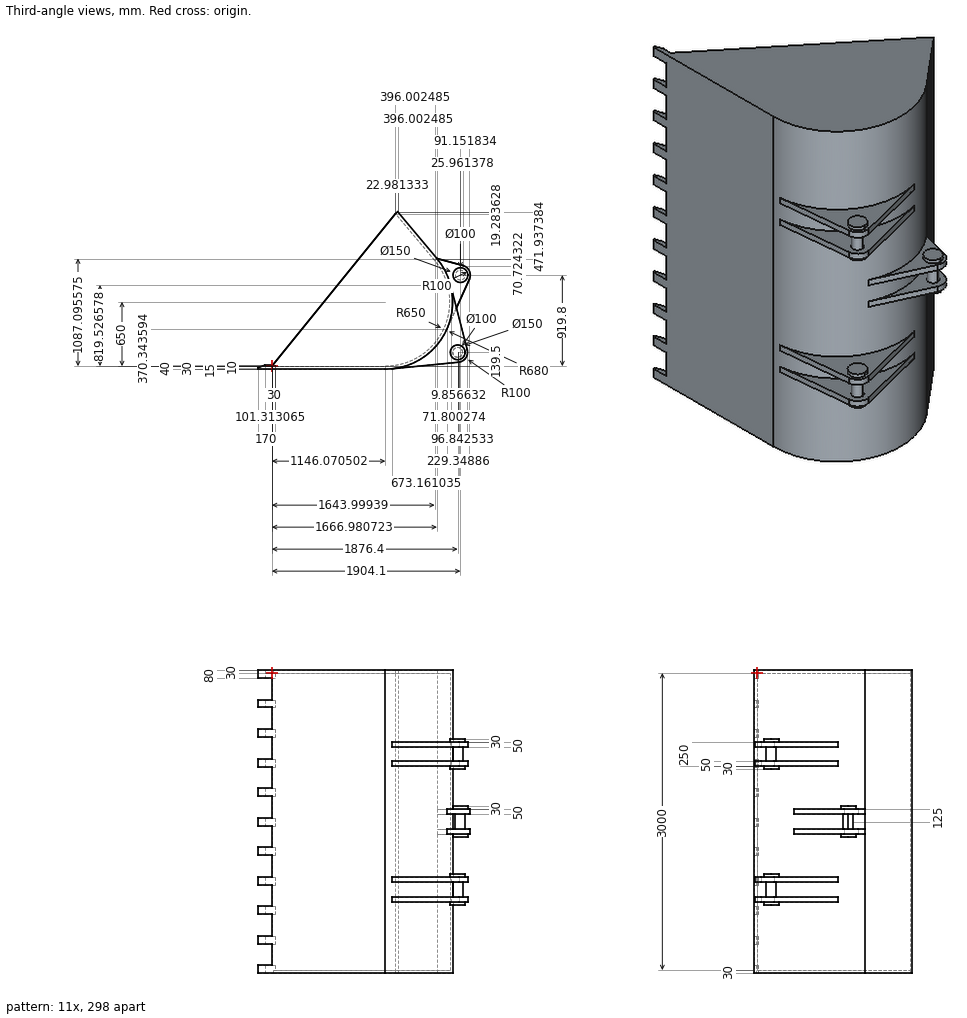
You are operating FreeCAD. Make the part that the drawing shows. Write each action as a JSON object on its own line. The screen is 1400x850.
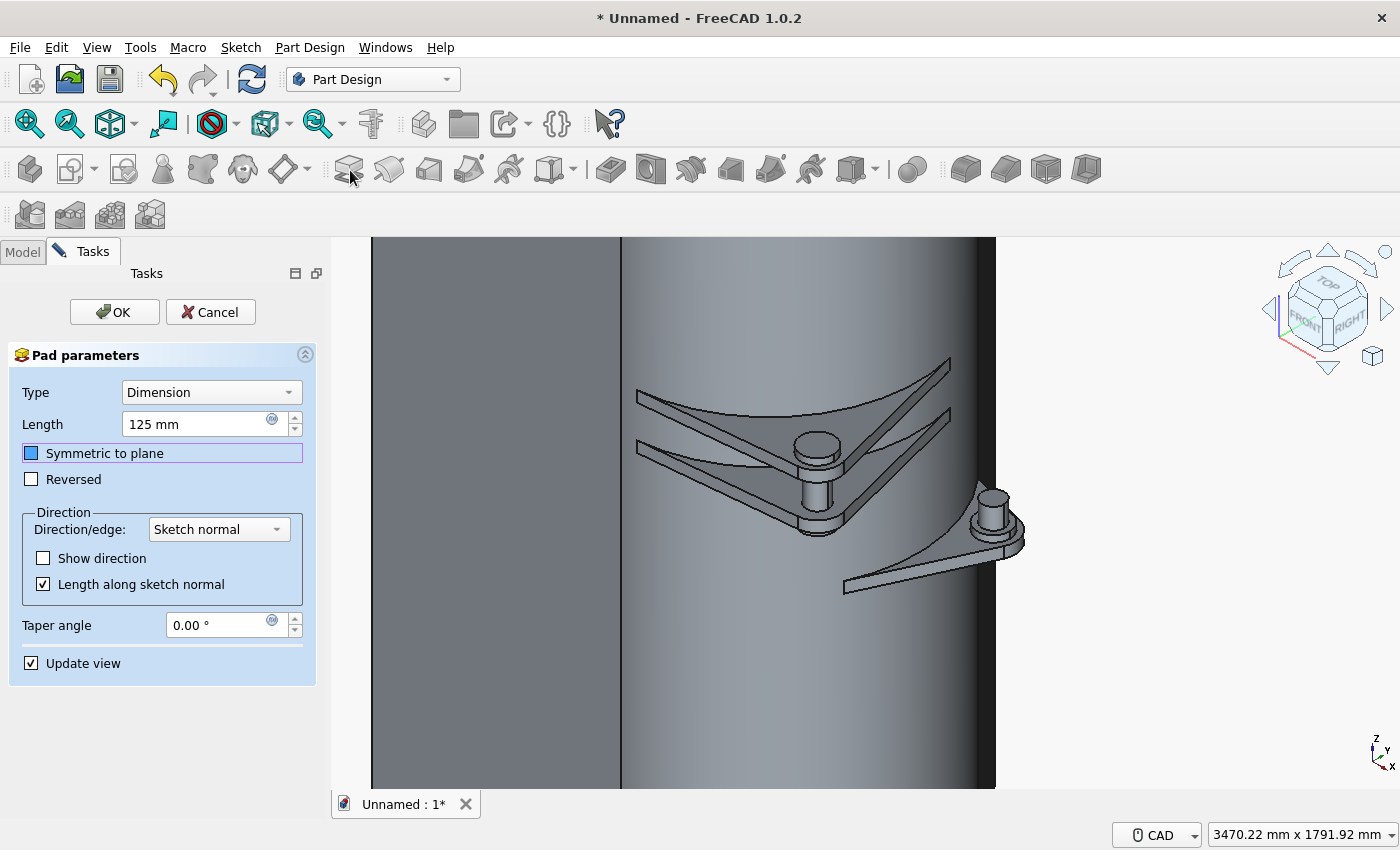
{"action": "left_click", "coordinate": [30, 479]}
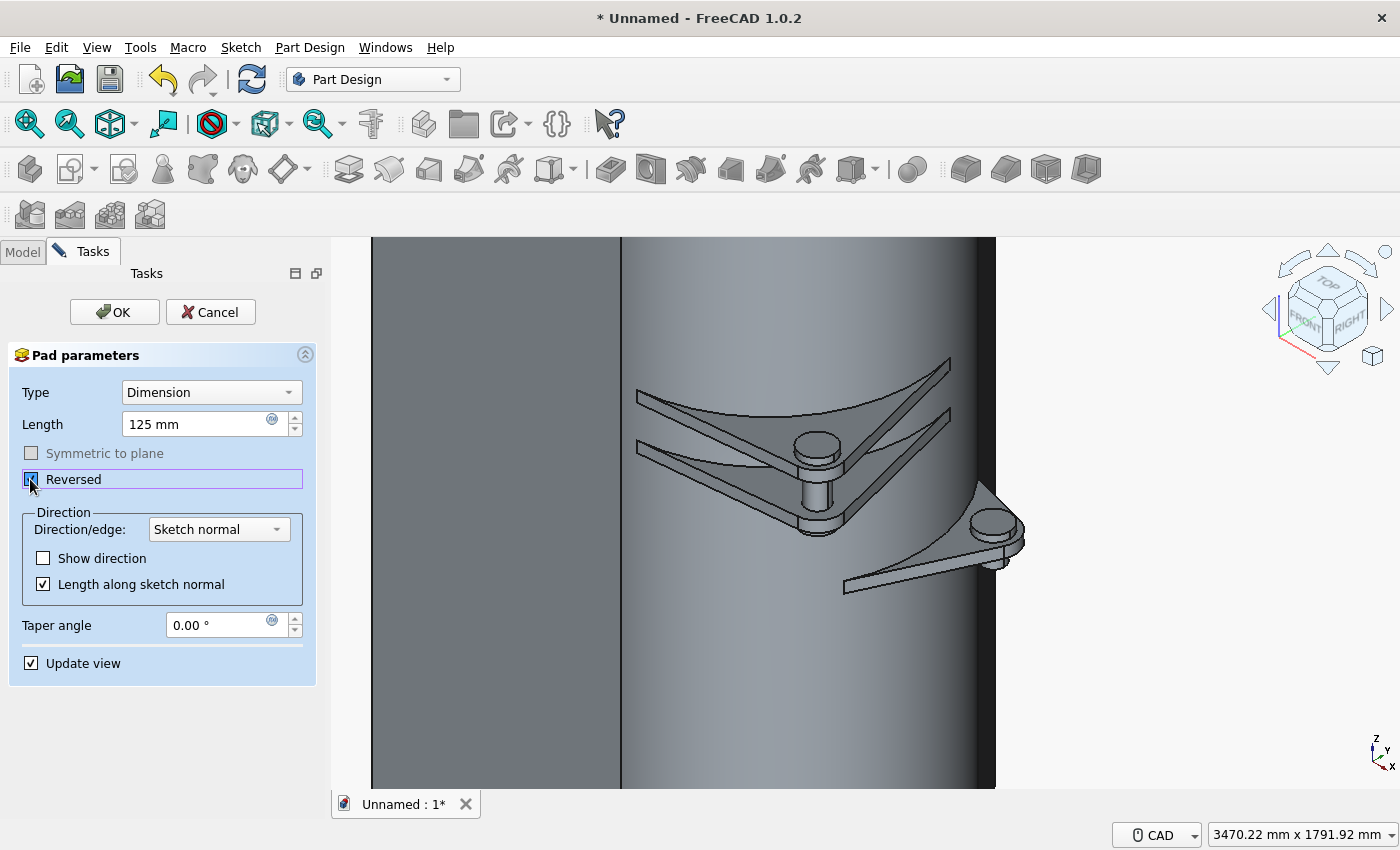
{"action": "left_click", "coordinate": [115, 312]}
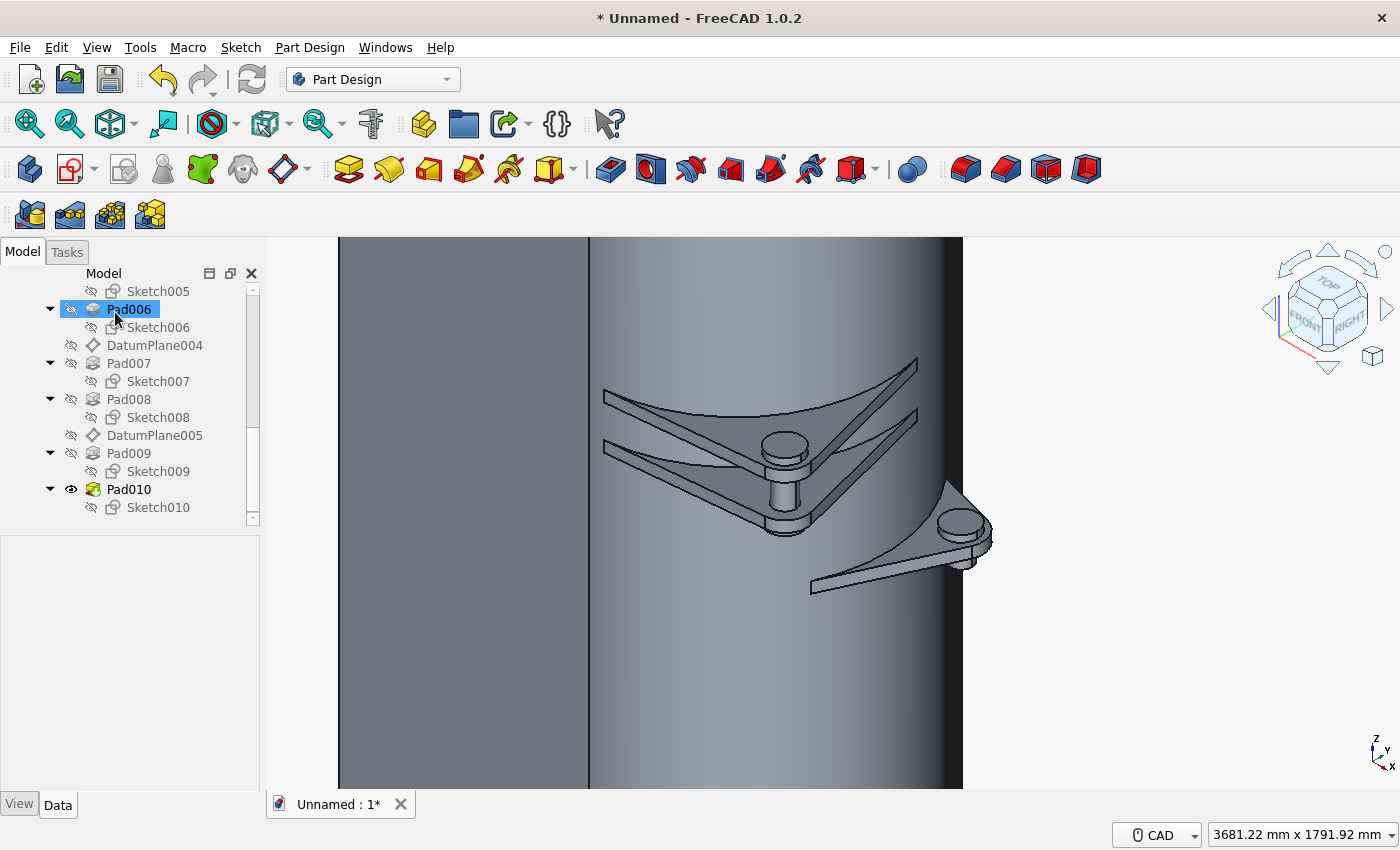
{"action": "key", "text": "v f"}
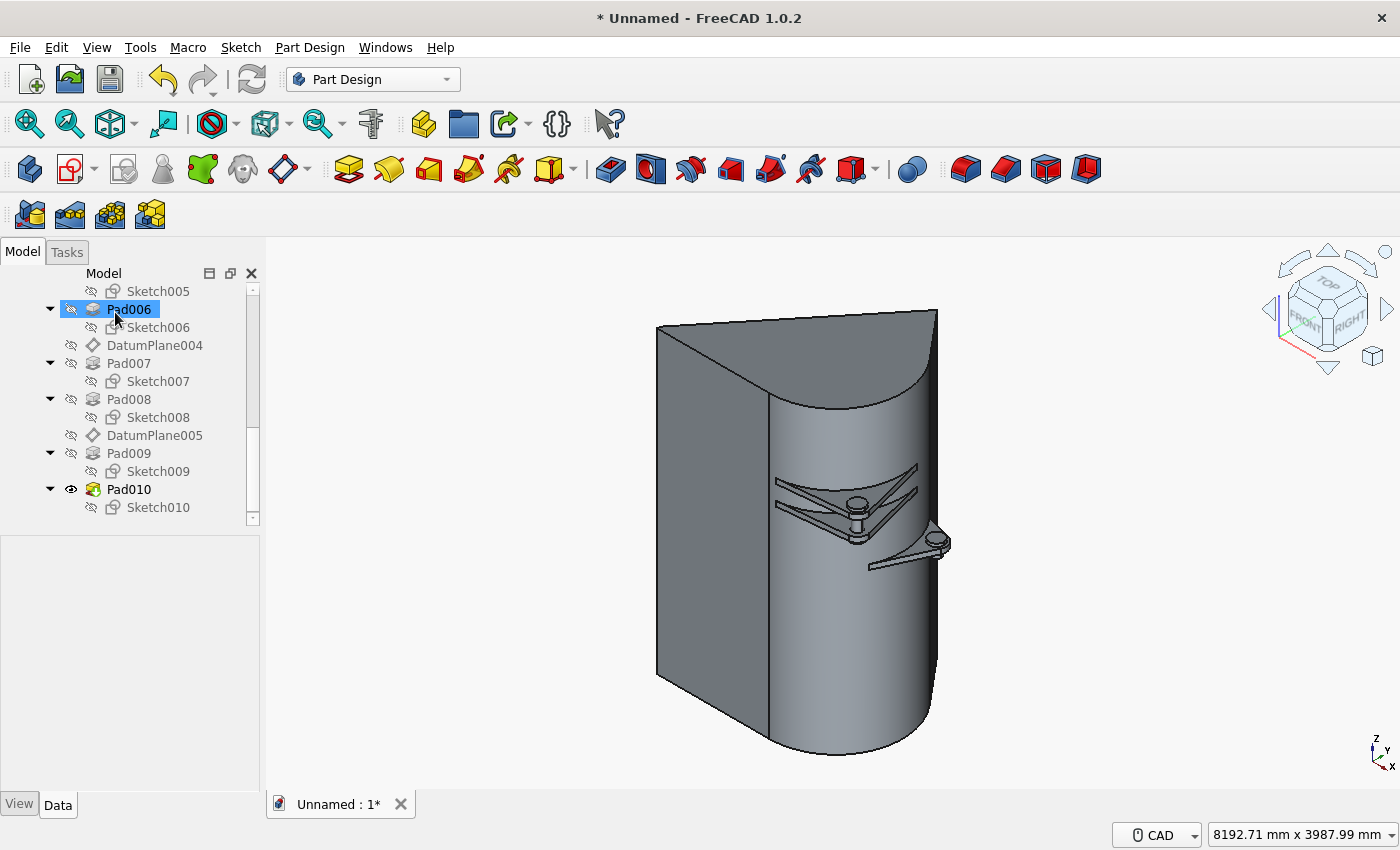
{"action": "scroll", "coordinate": [160, 395], "scroll_direction": "down", "scroll_amount": 3}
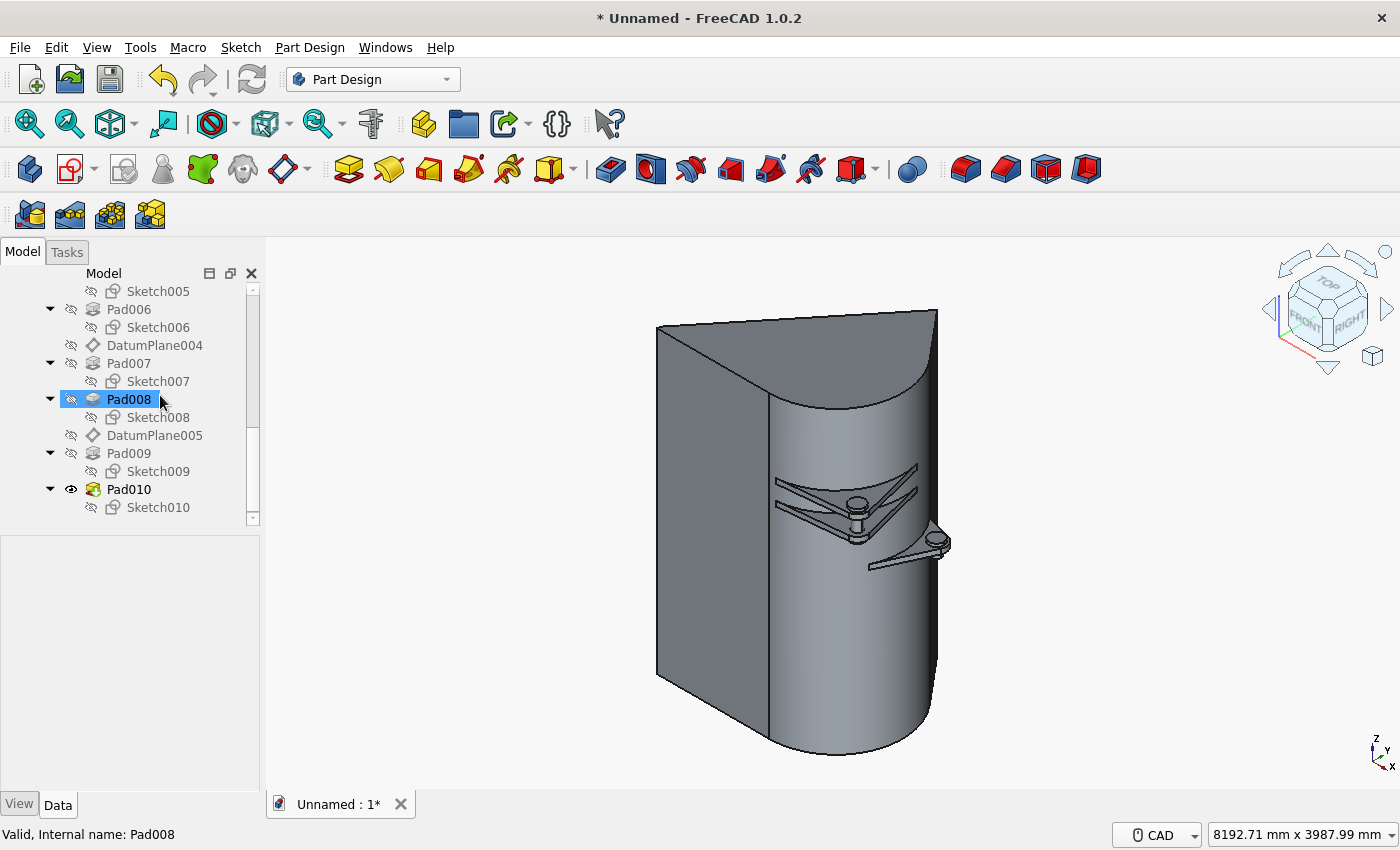
{"action": "scroll", "coordinate": [160, 395], "scroll_direction": "up", "scroll_amount": 15}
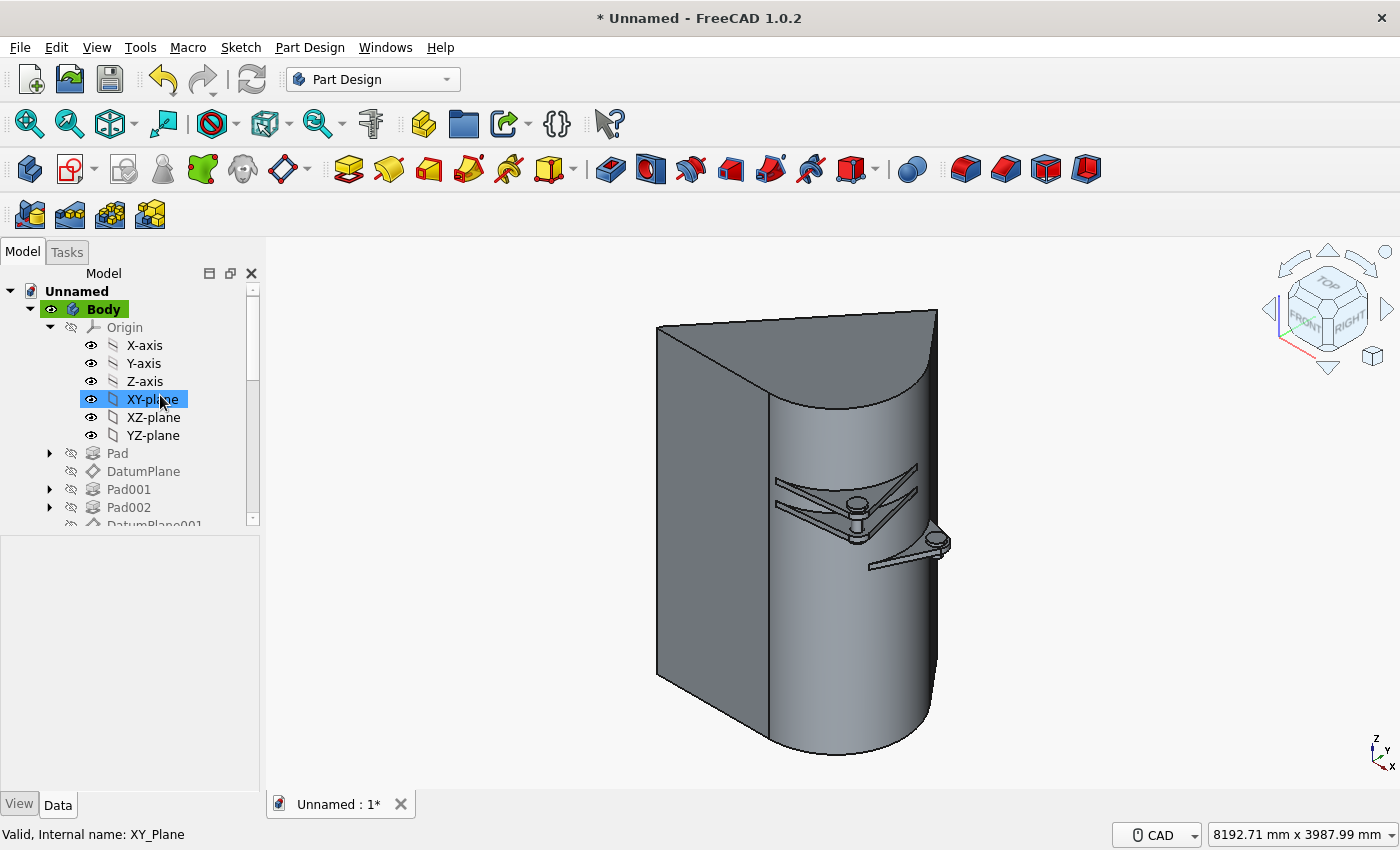
{"action": "left_click", "coordinate": [136, 399]}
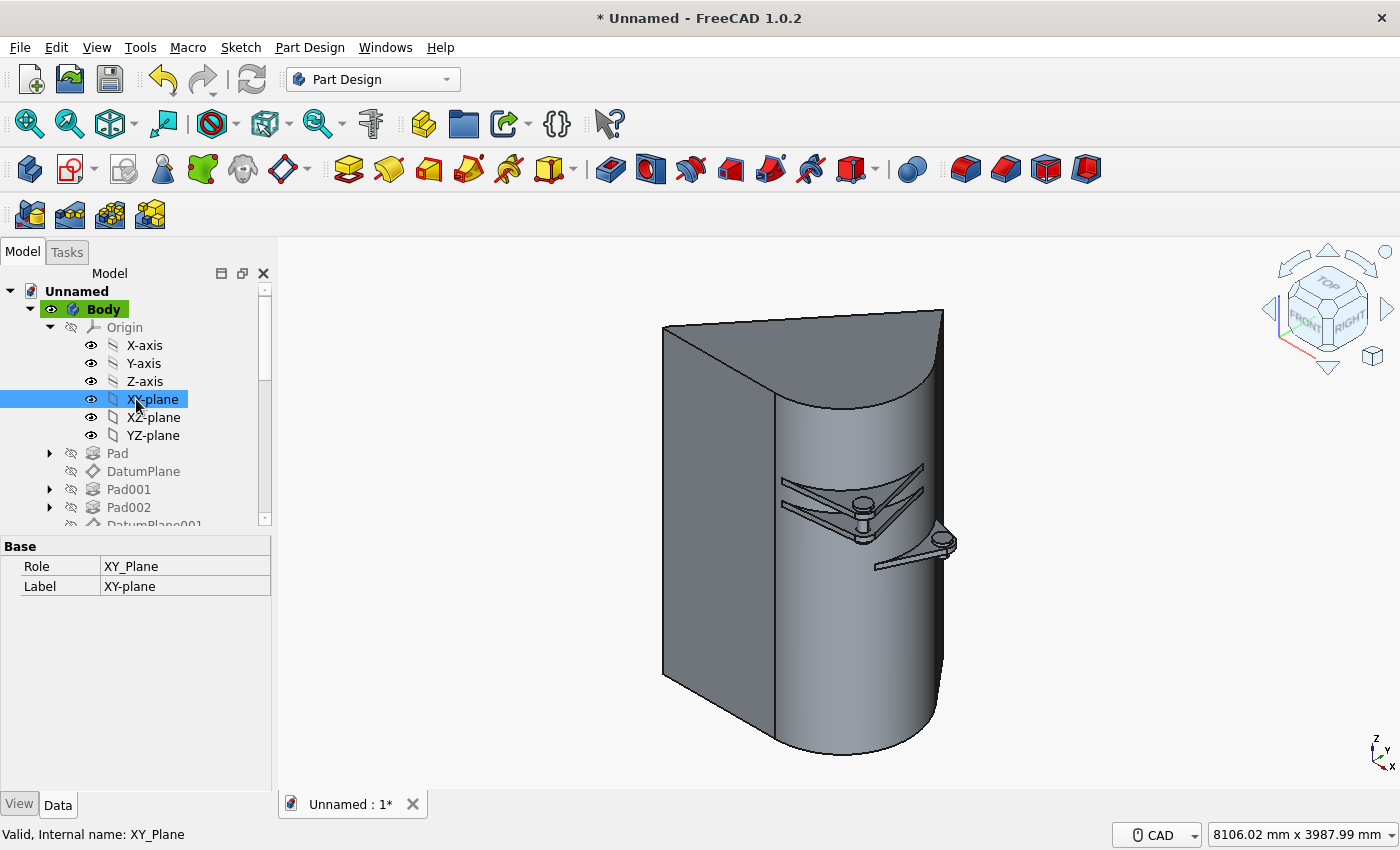
{"action": "left_click", "coordinate": [284, 170]}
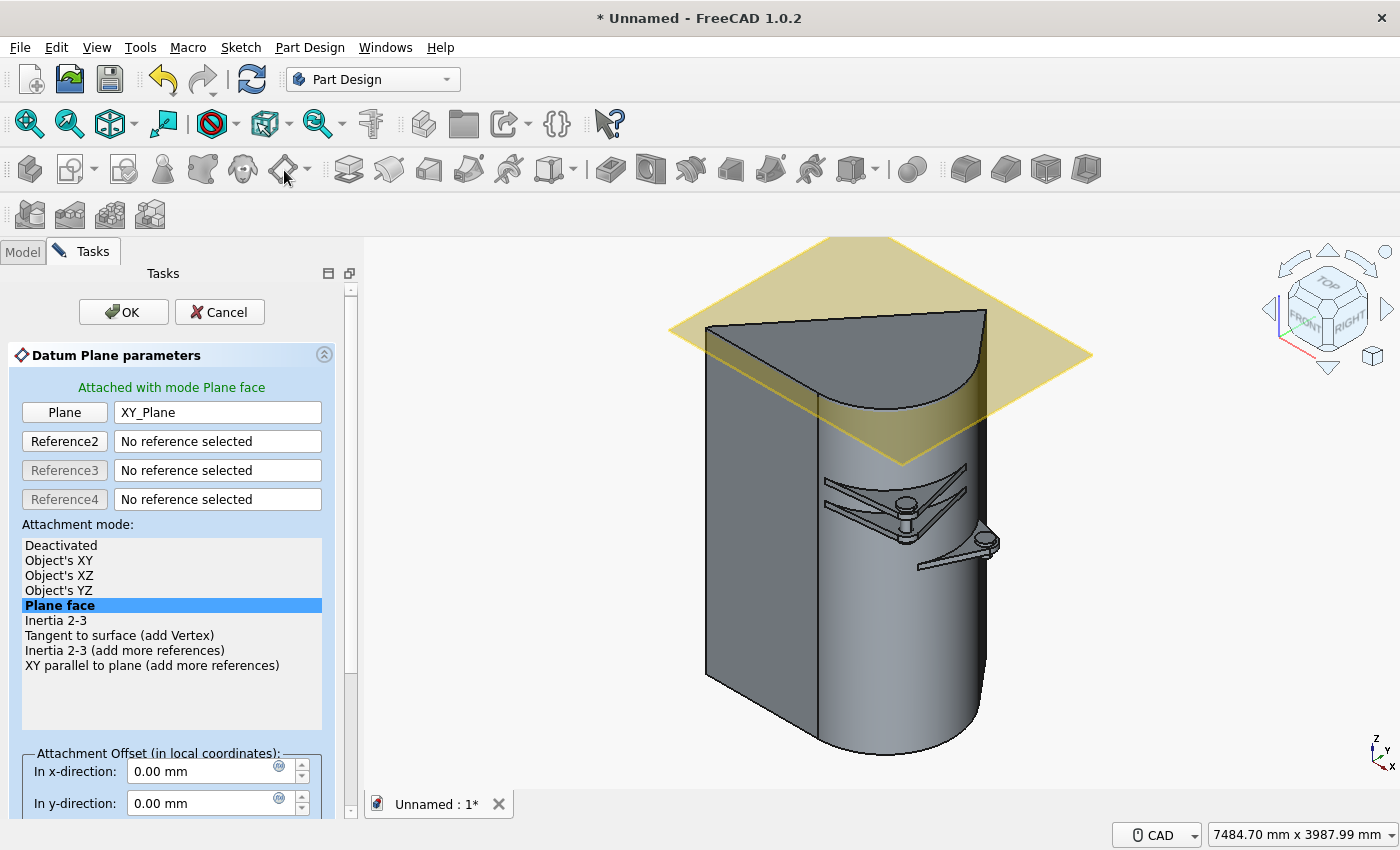
{"action": "scroll", "coordinate": [351, 550], "scroll_direction": "down", "scroll_amount": 2}